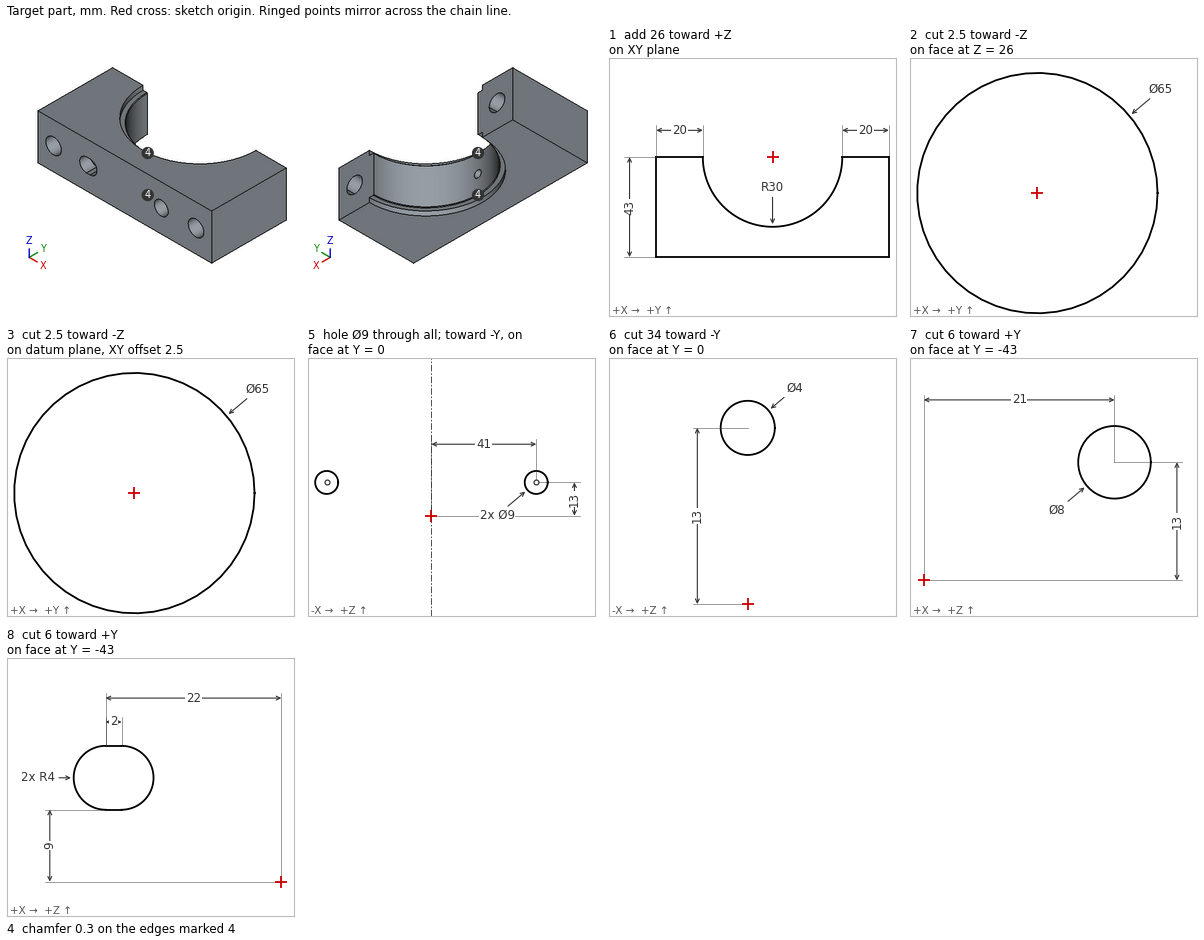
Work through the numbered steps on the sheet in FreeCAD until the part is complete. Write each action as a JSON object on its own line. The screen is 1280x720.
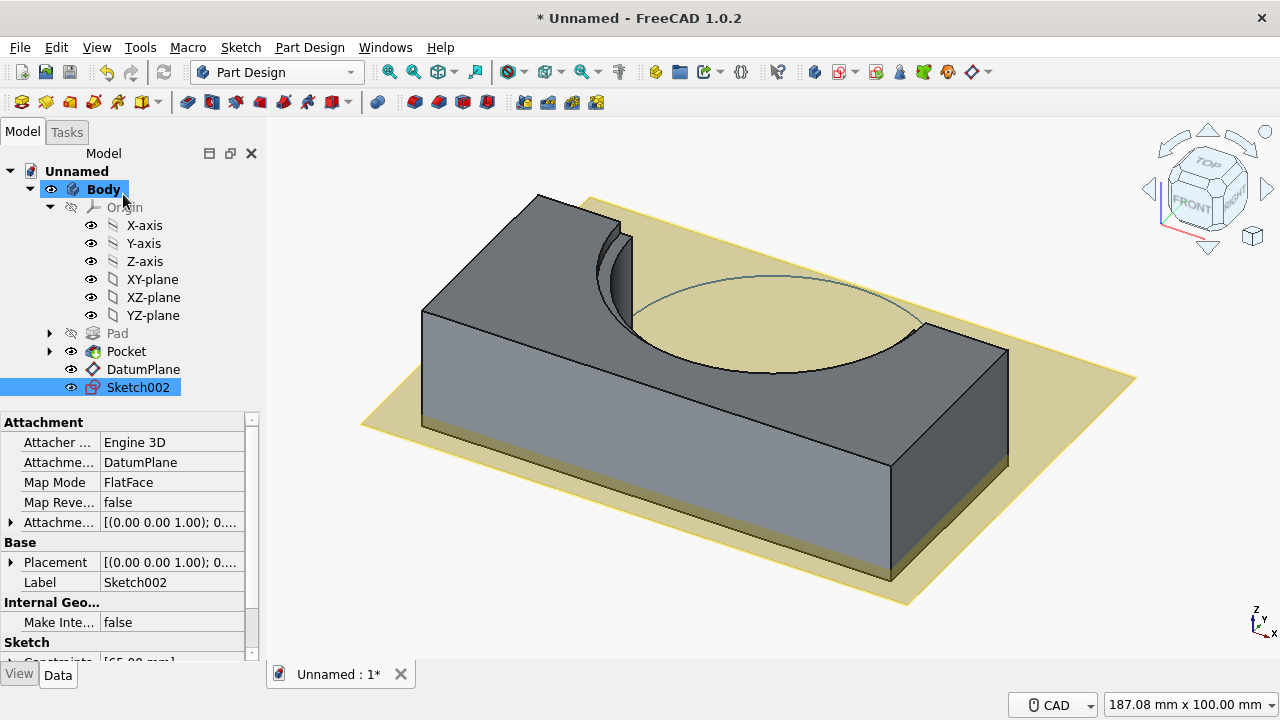
{"action": "left_click", "coordinate": [188, 102]}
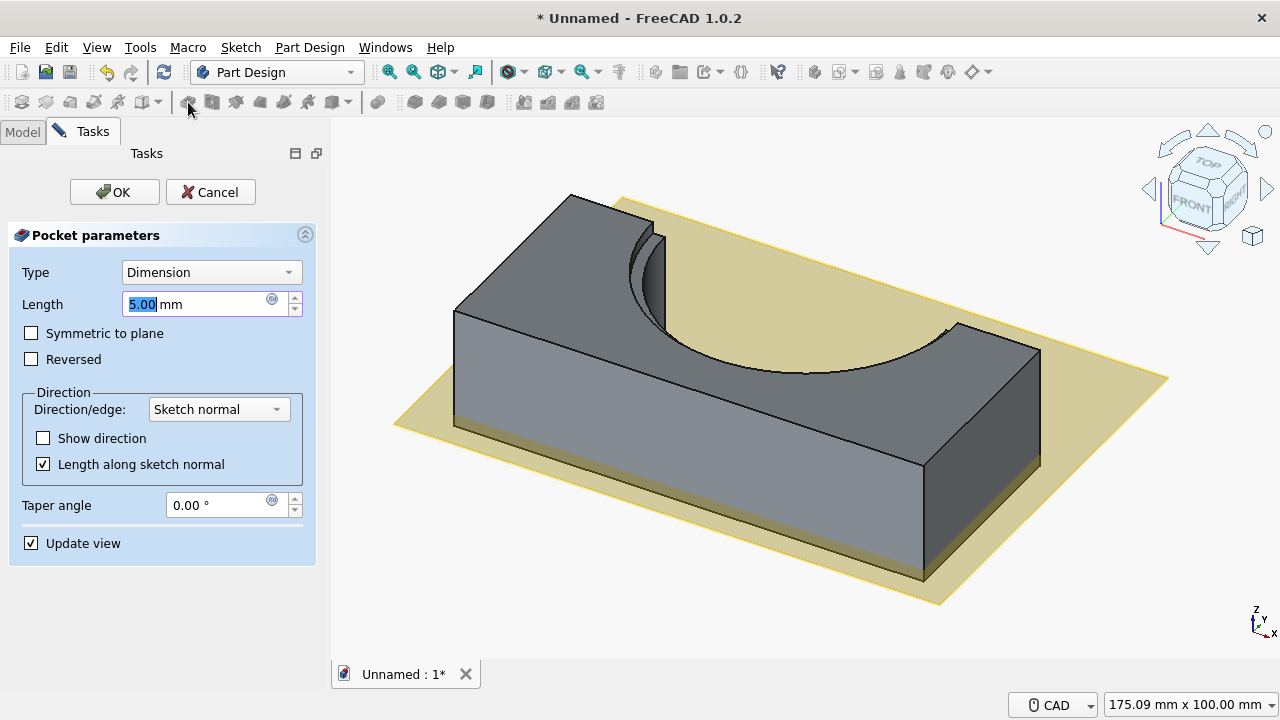
{"action": "type", "text": "2.5"}
{"action": "key", "text": "Tab"}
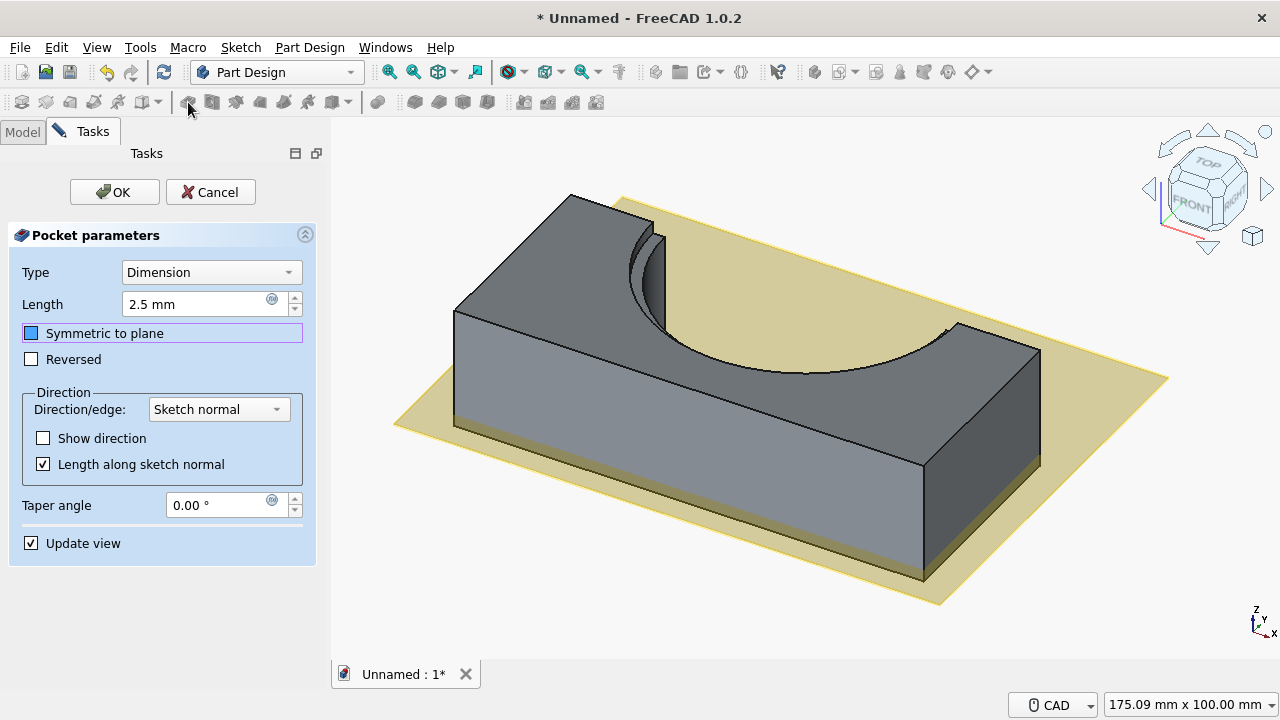
{"action": "left_click", "coordinate": [115, 192]}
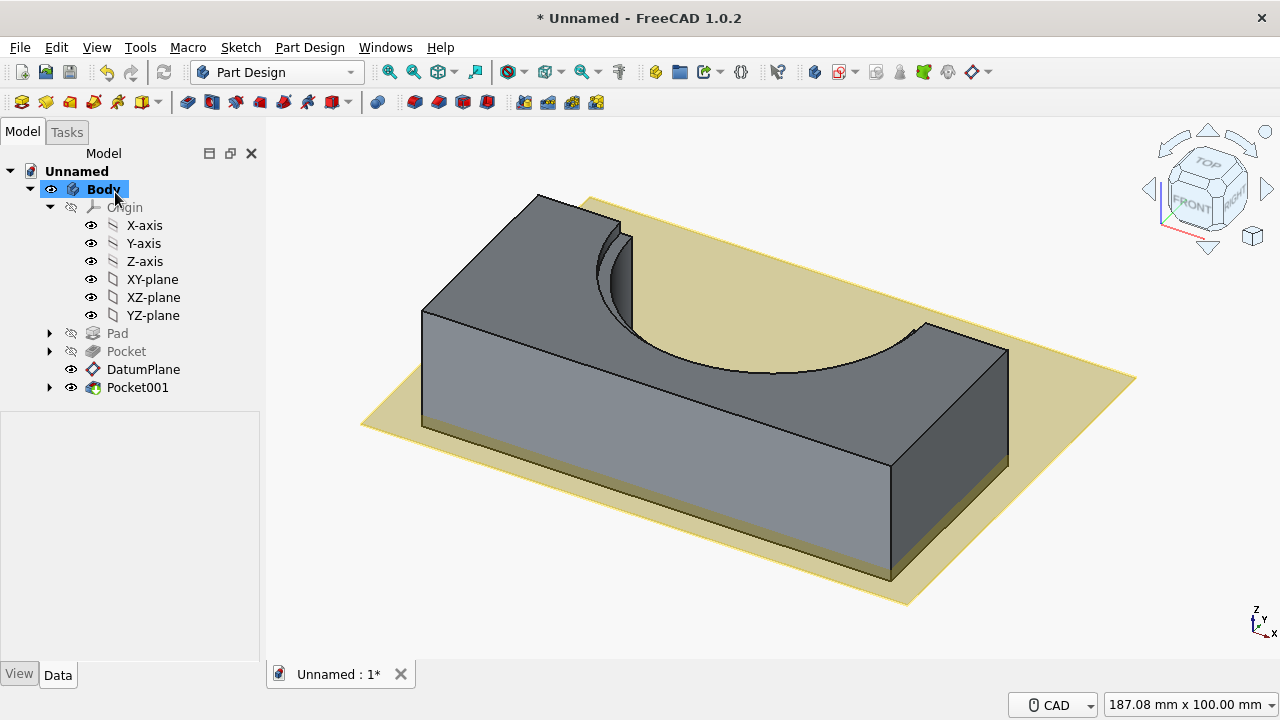
{"action": "left_click", "coordinate": [116, 369]}
{"action": "key", "text": "space"}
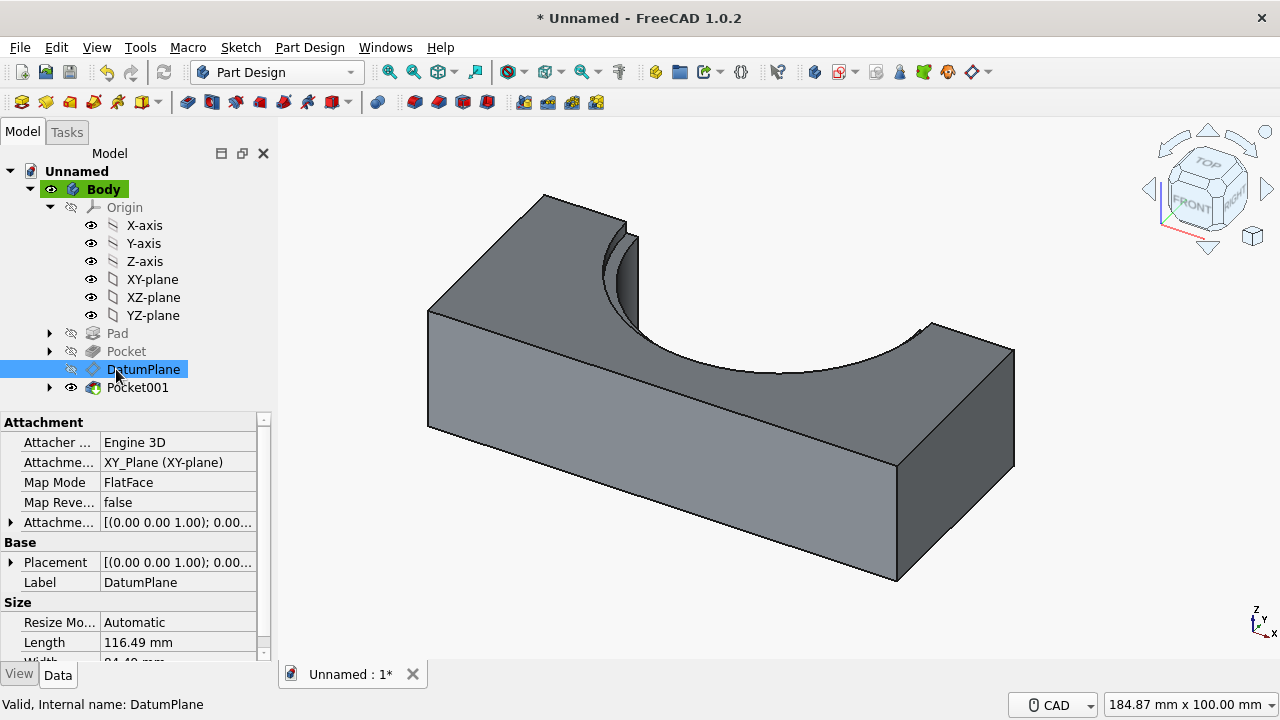
{"action": "left_click", "coordinate": [618, 269]}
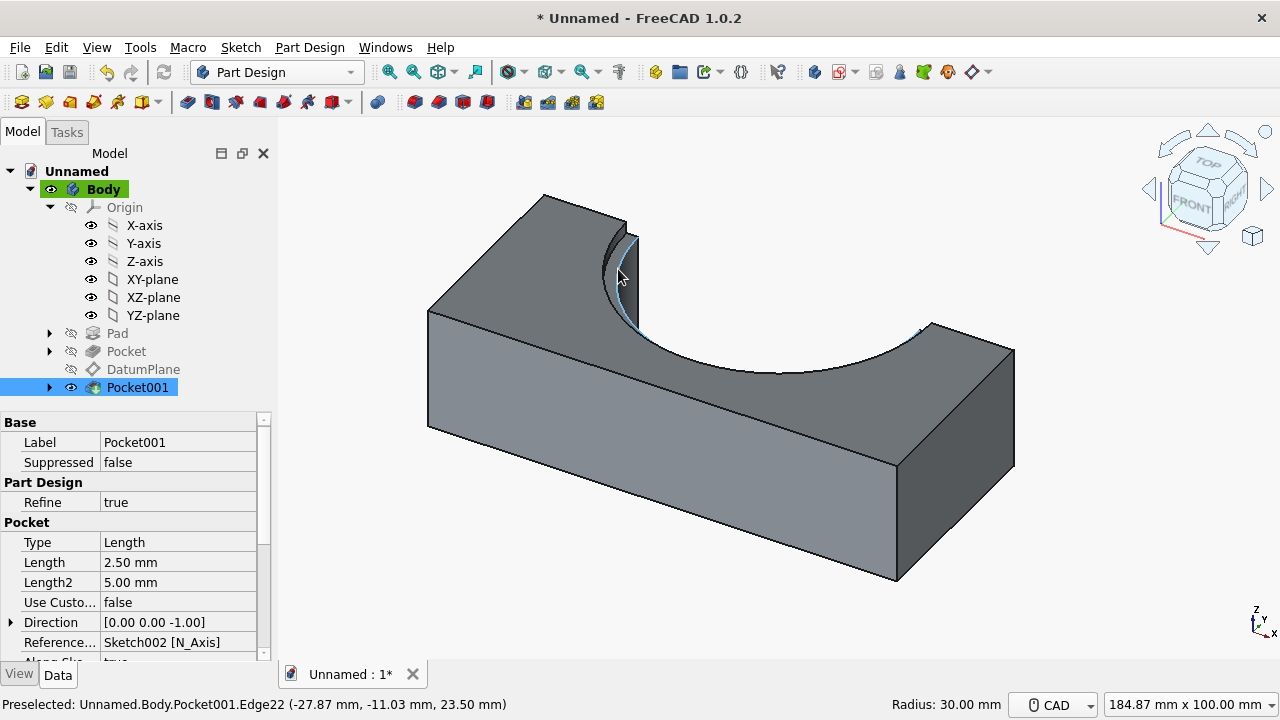
{"action": "key", "text": "0"}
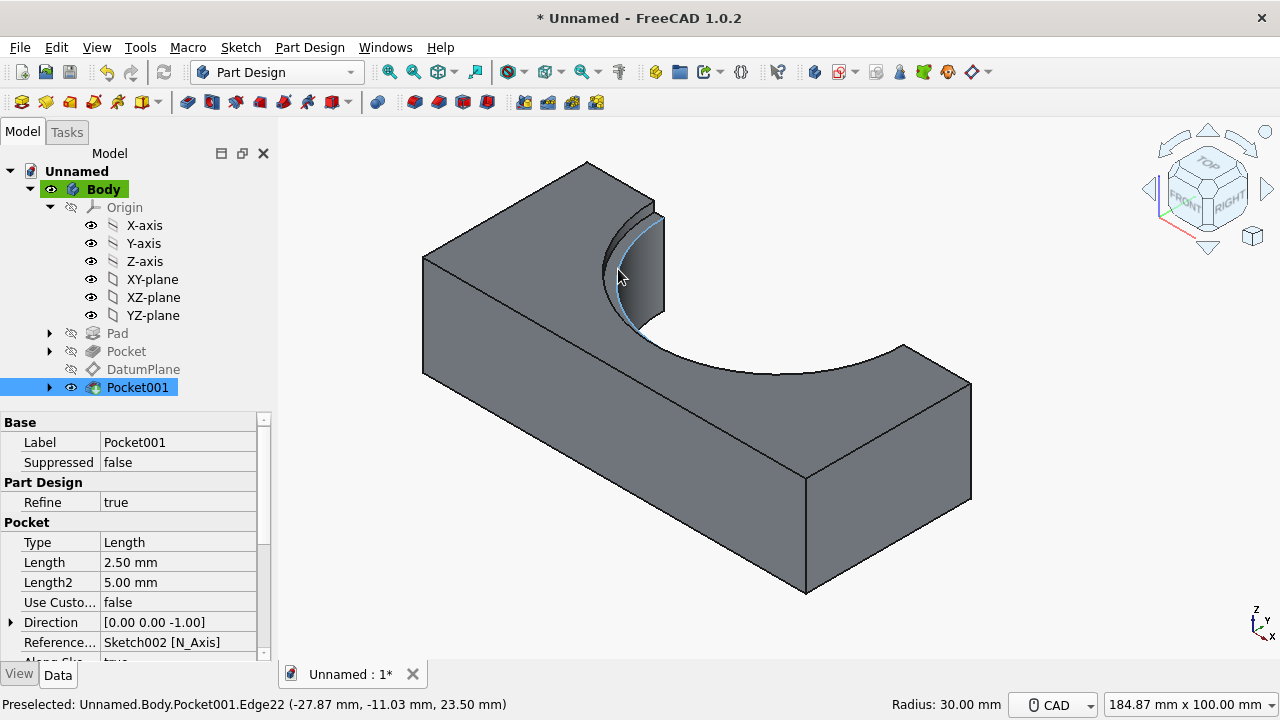
{"action": "key", "text": "2"}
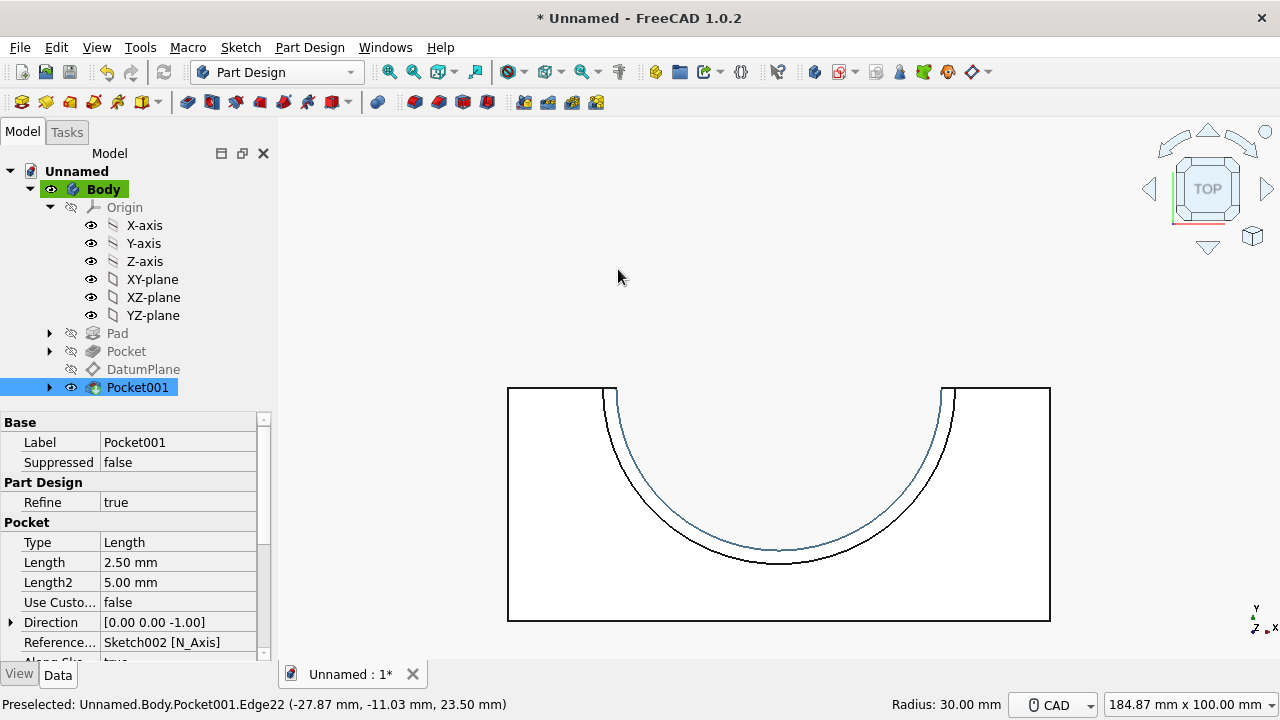
{"action": "key", "text": "1"}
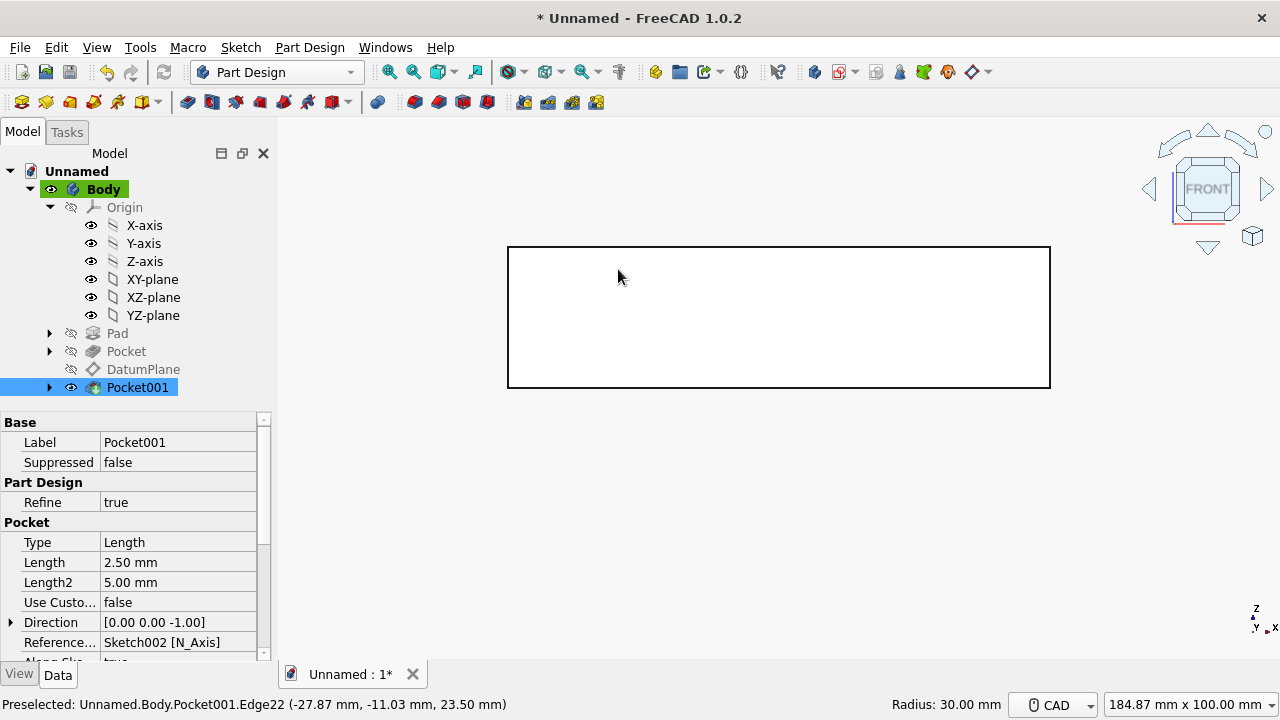
{"action": "key", "text": "3"}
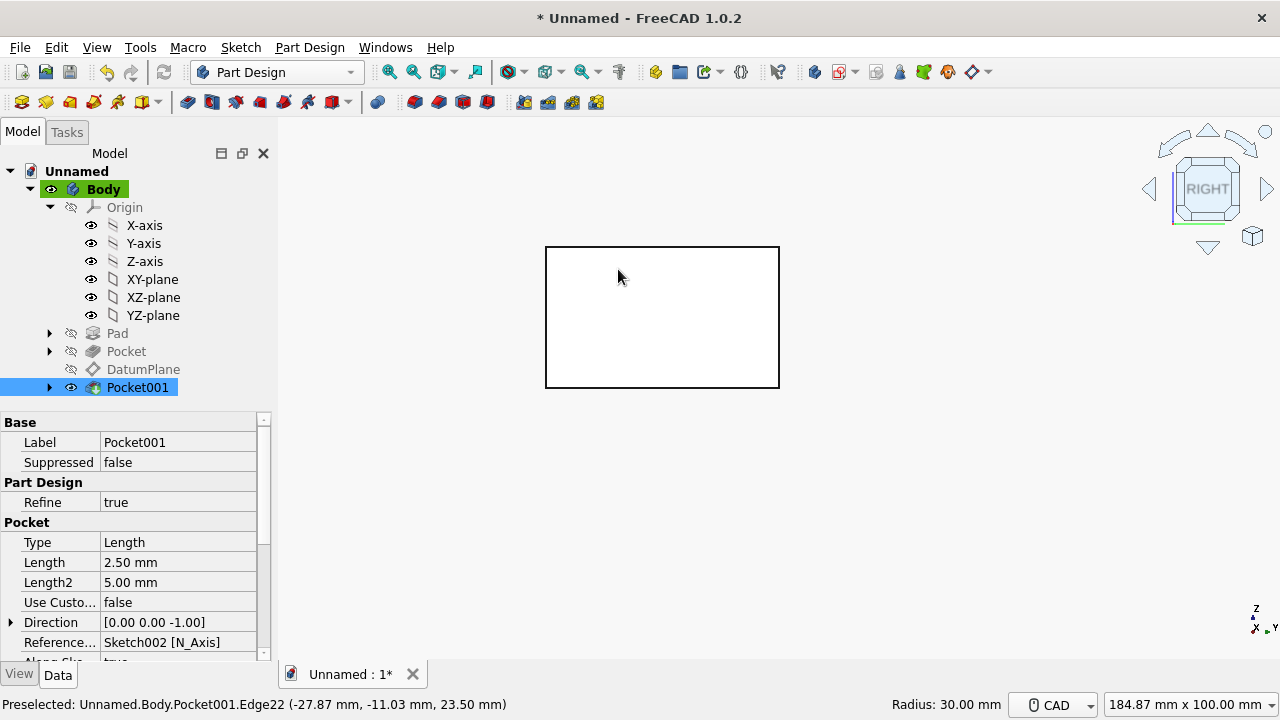
{"action": "left_click", "coordinate": [390, 72]}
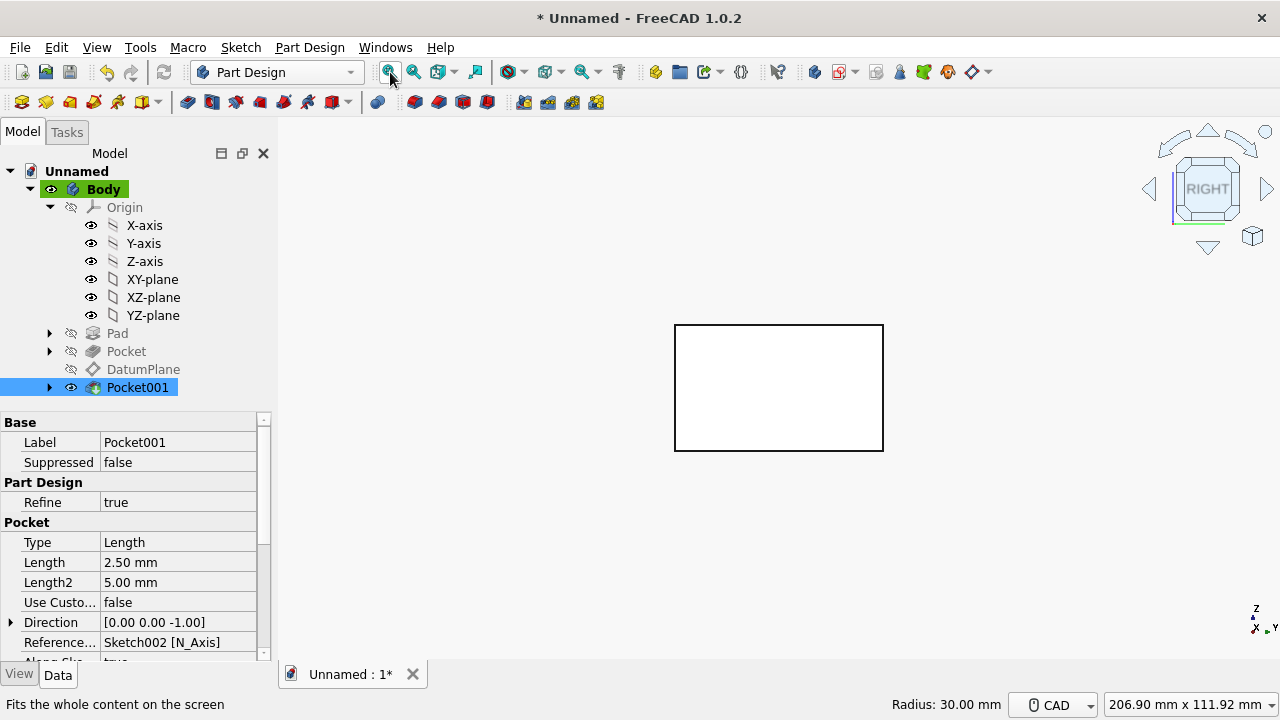
{"action": "key", "text": "5"}